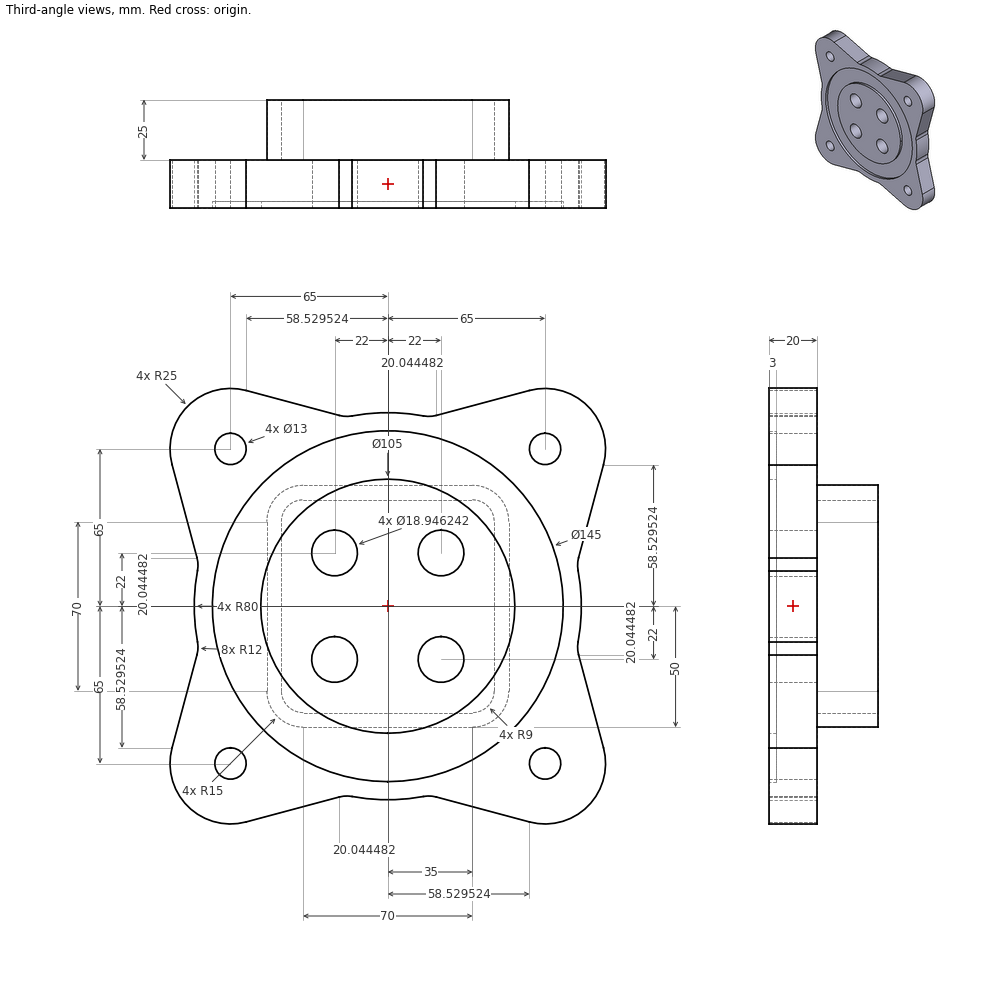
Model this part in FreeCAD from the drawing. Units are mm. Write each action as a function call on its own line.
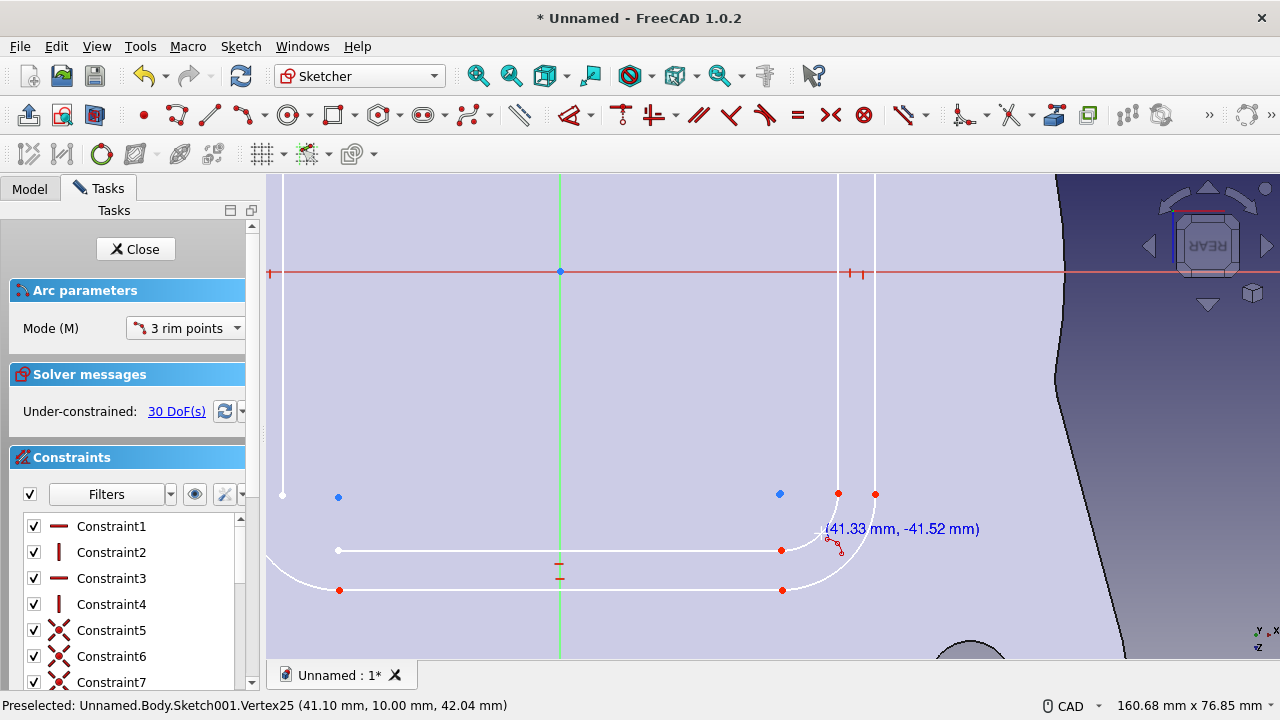
click(338, 551)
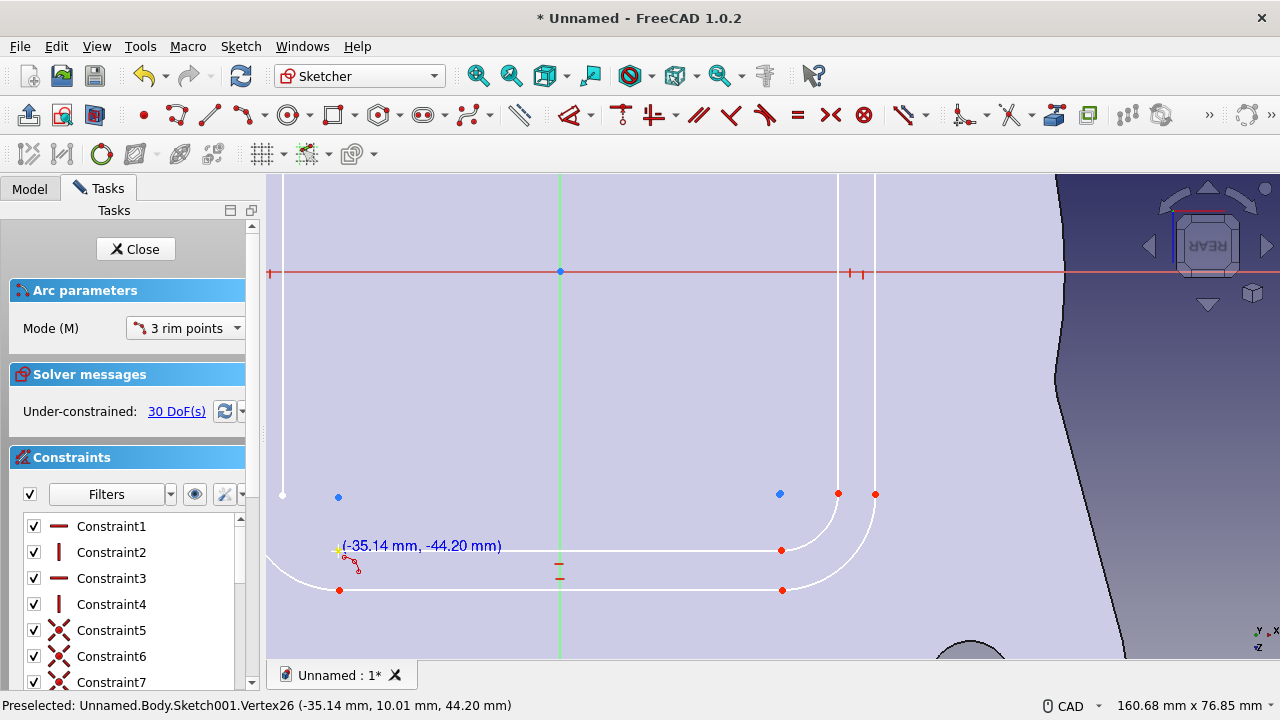
scroll(822, 534, down, 4)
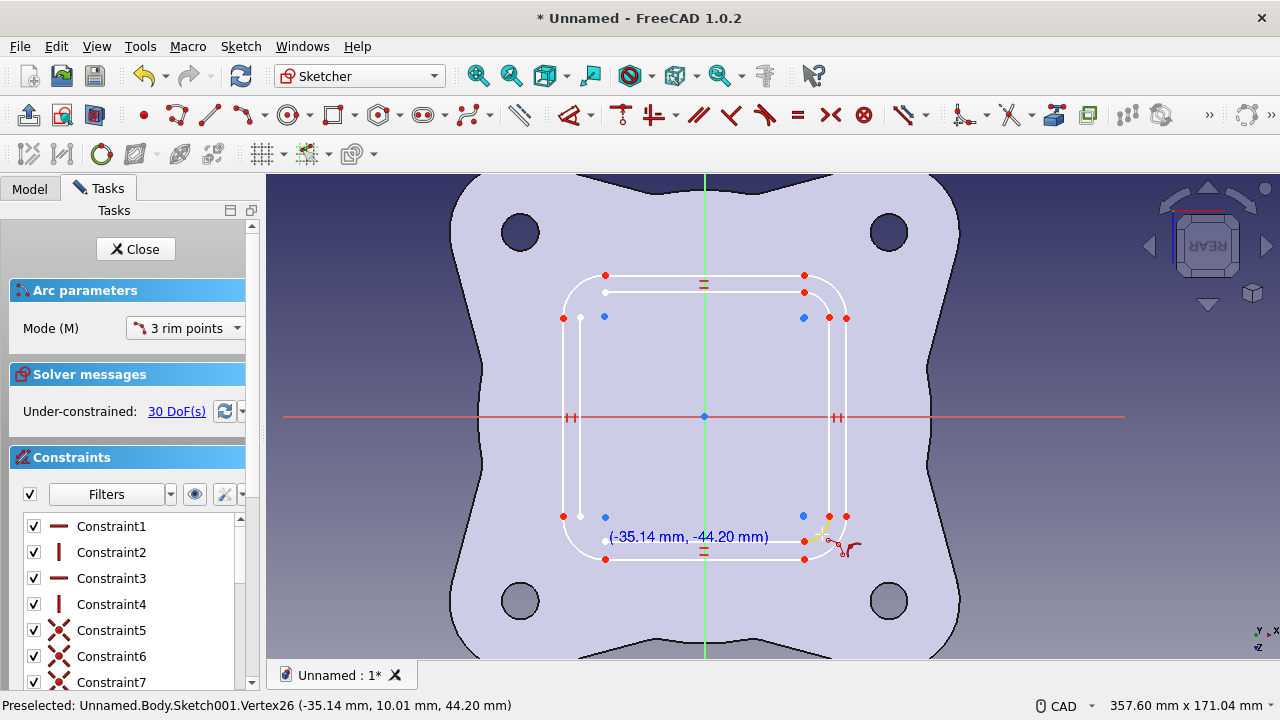
click(580, 517)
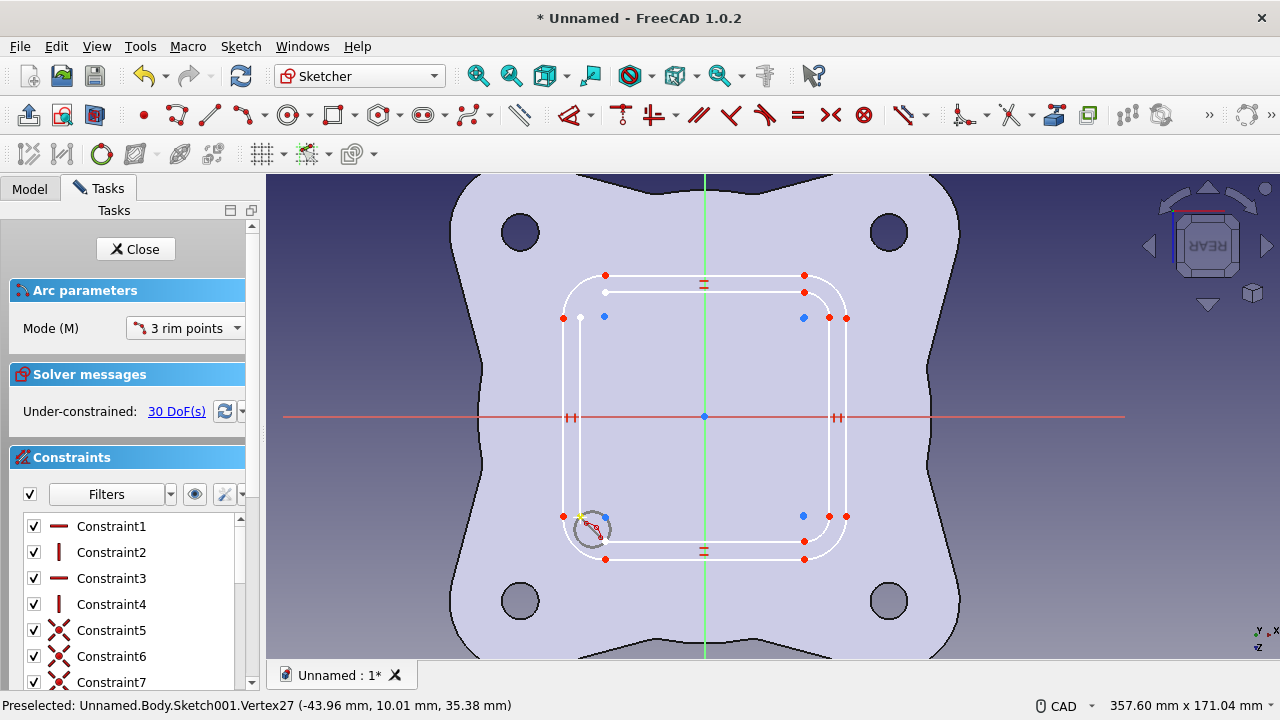
scroll(587, 534, up, 4)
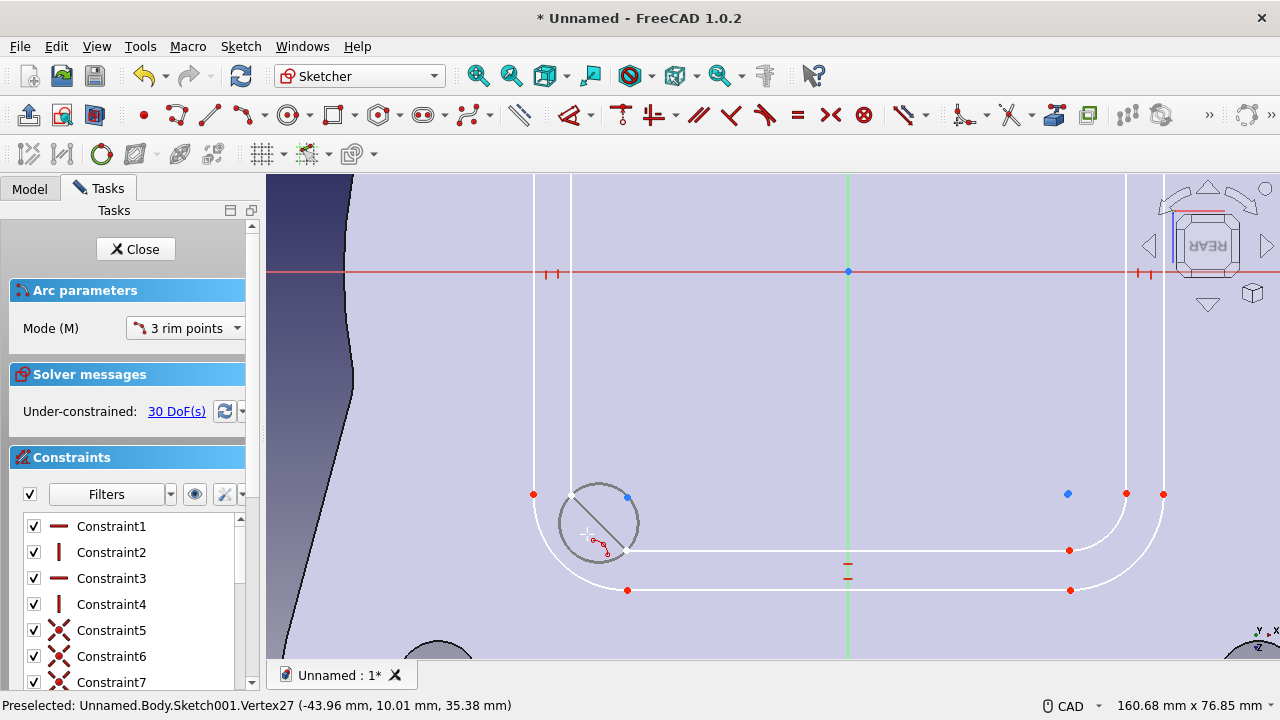
click(587, 533)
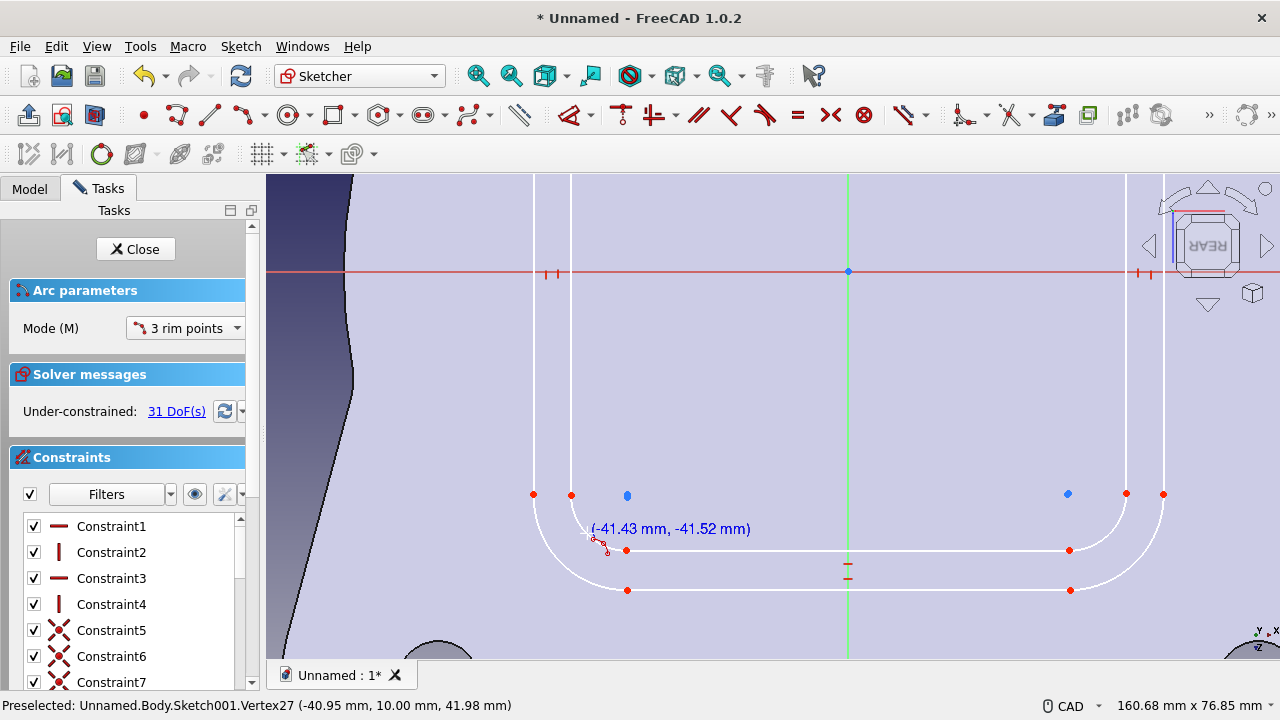
scroll(587, 534, down, 4)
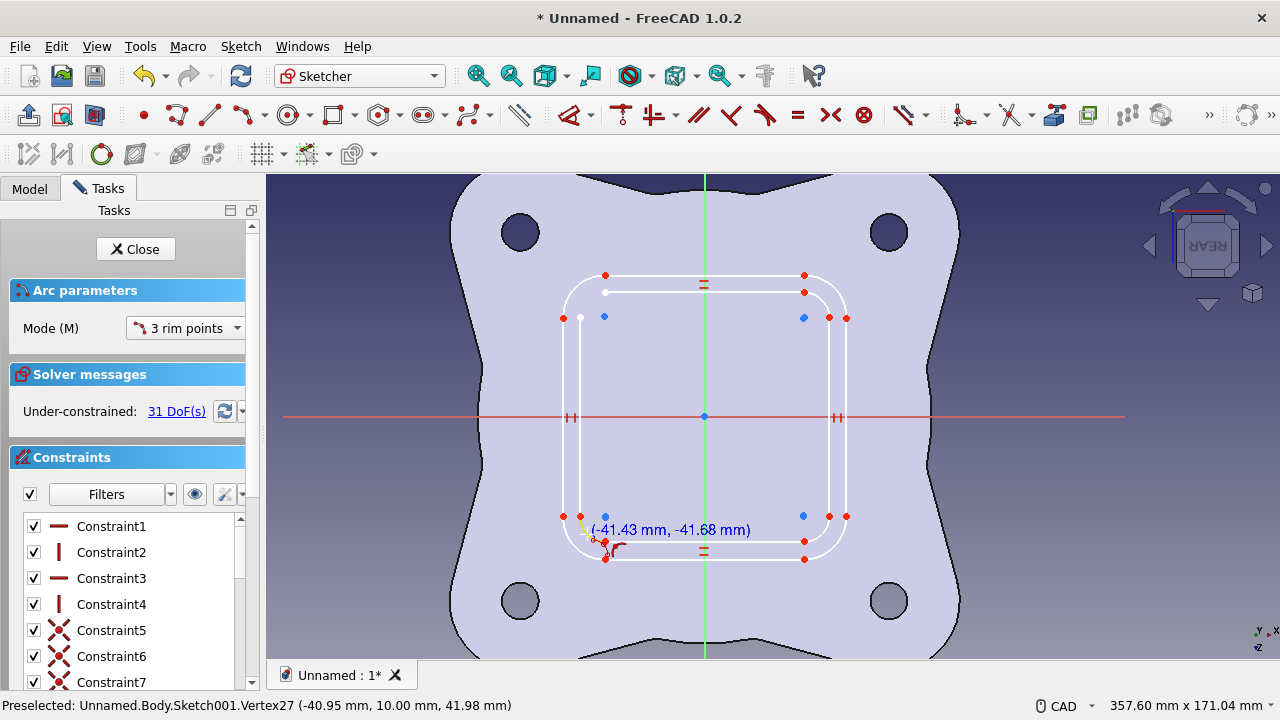
click(580, 318)
click(606, 292)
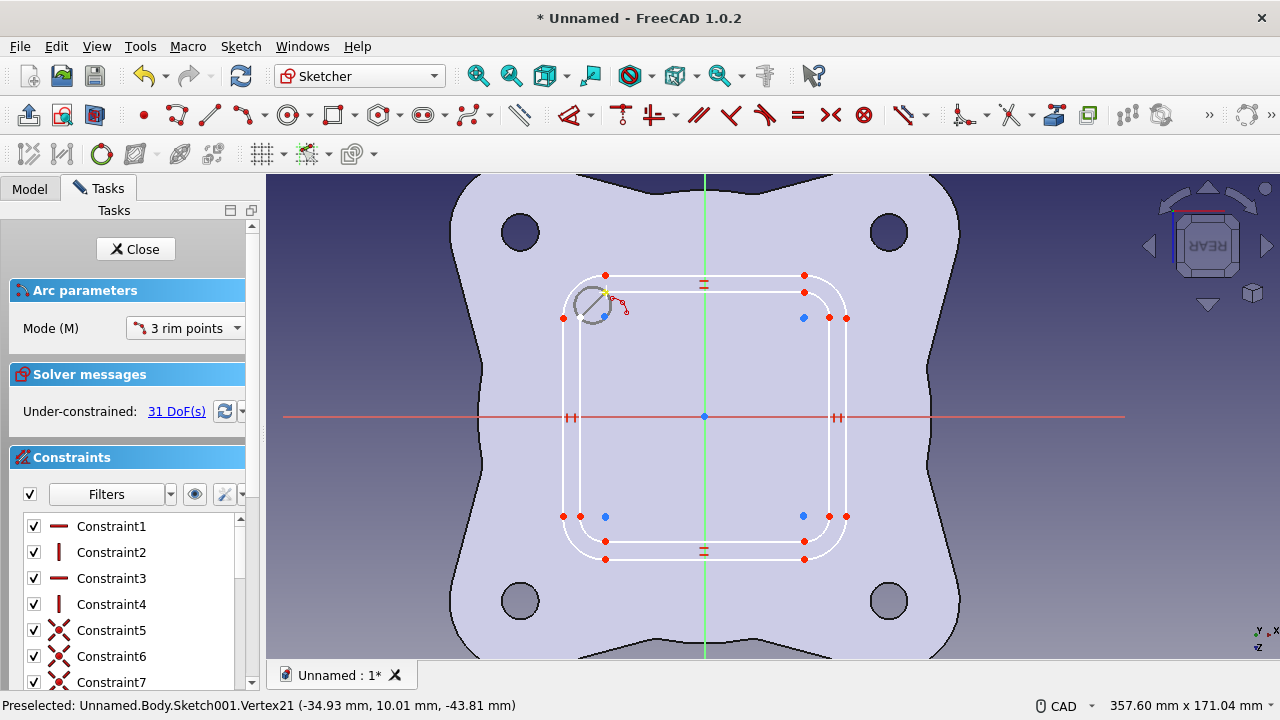
scroll(587, 299, up, 4)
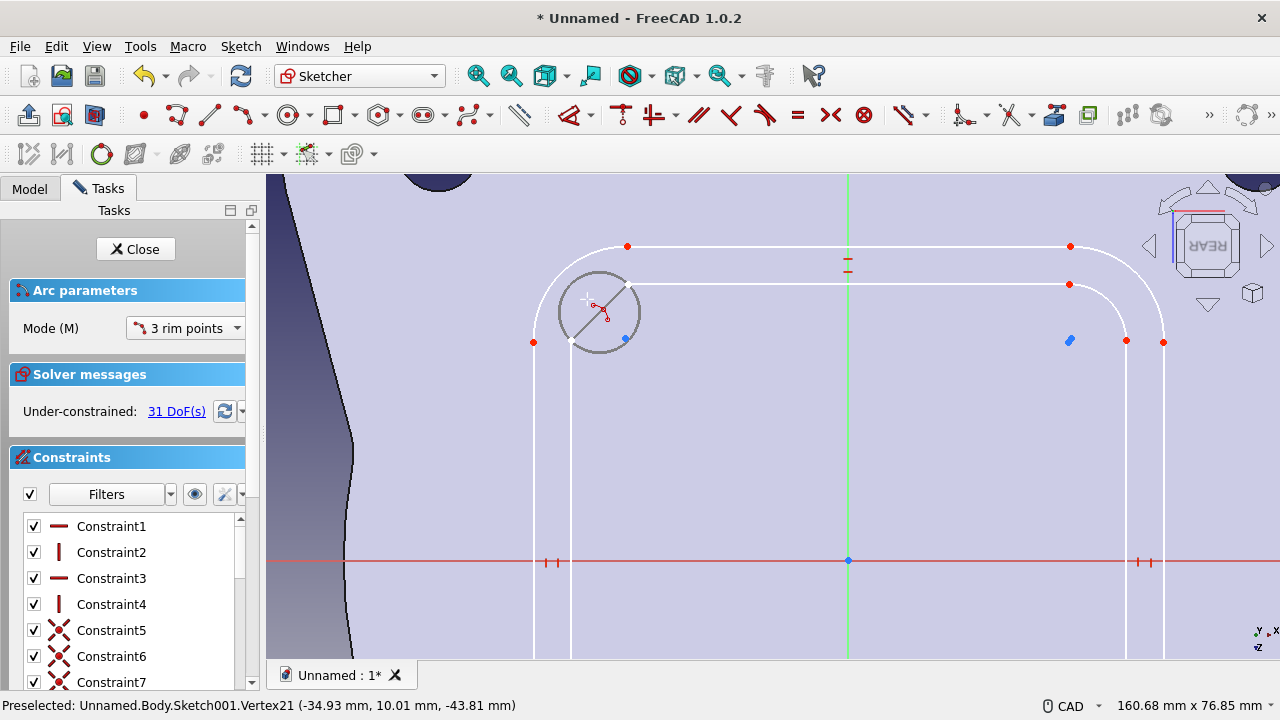
click(587, 300)
key(Escape)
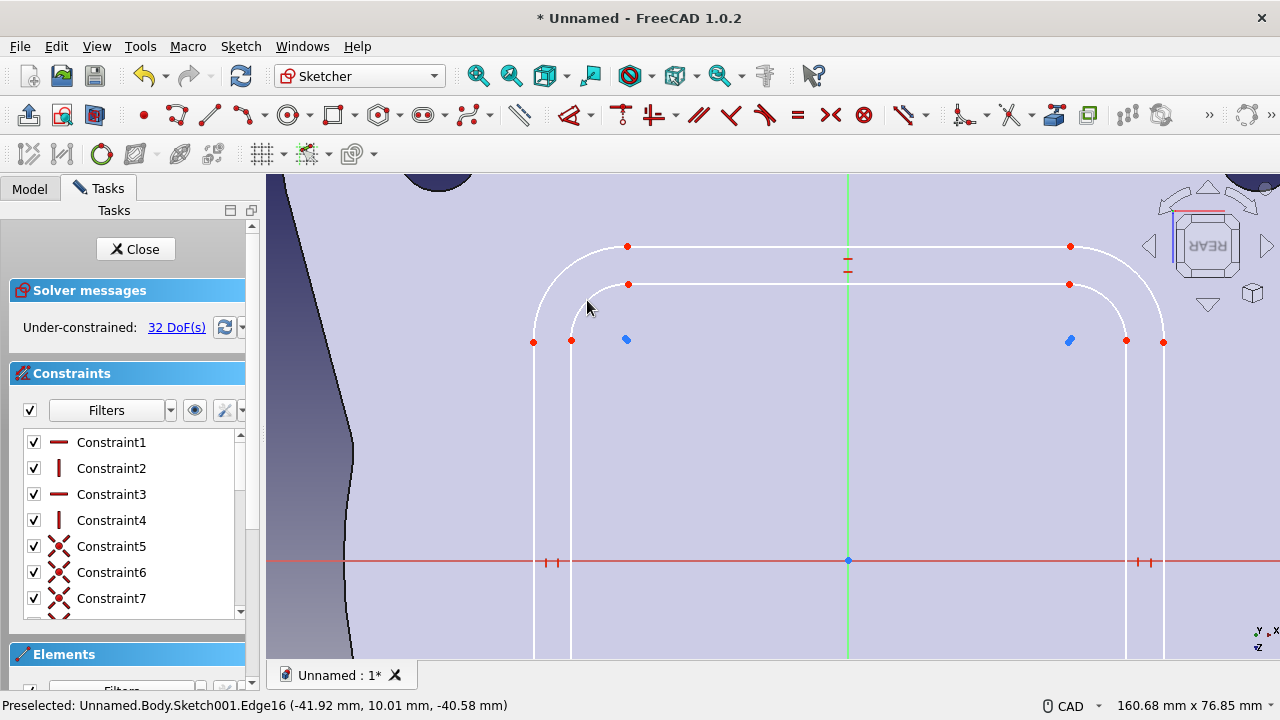
click(937, 247)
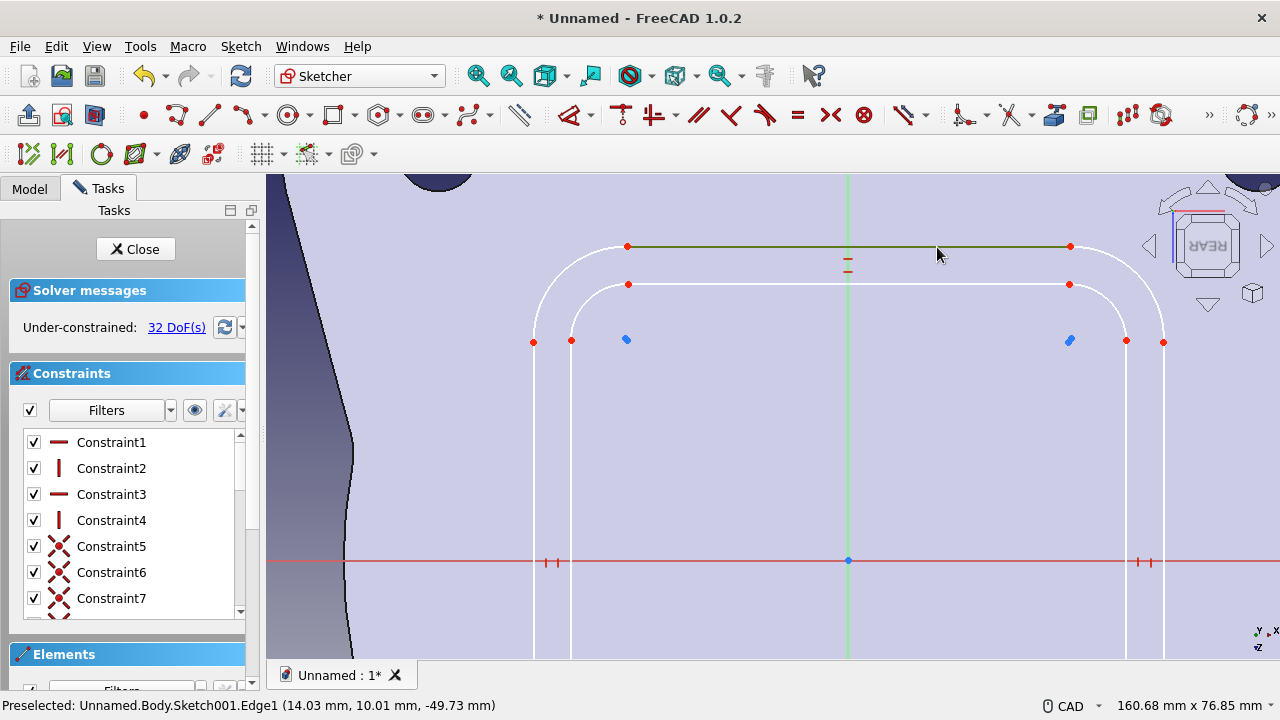
click(584, 257)